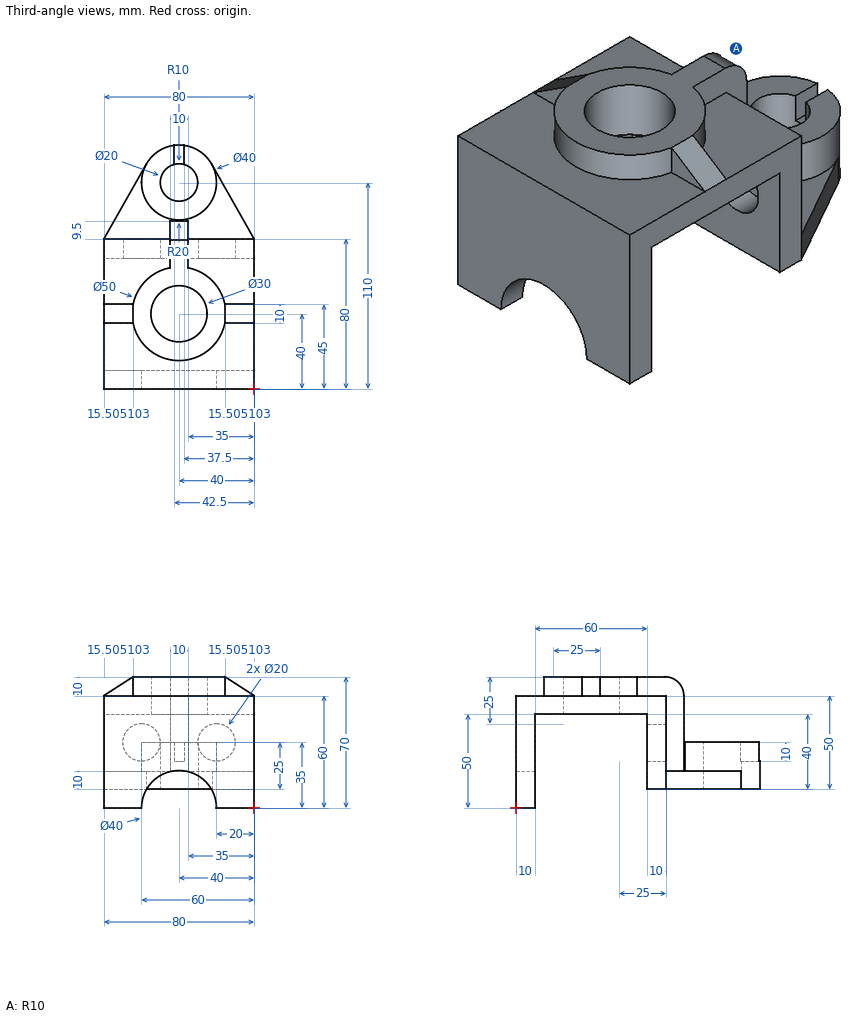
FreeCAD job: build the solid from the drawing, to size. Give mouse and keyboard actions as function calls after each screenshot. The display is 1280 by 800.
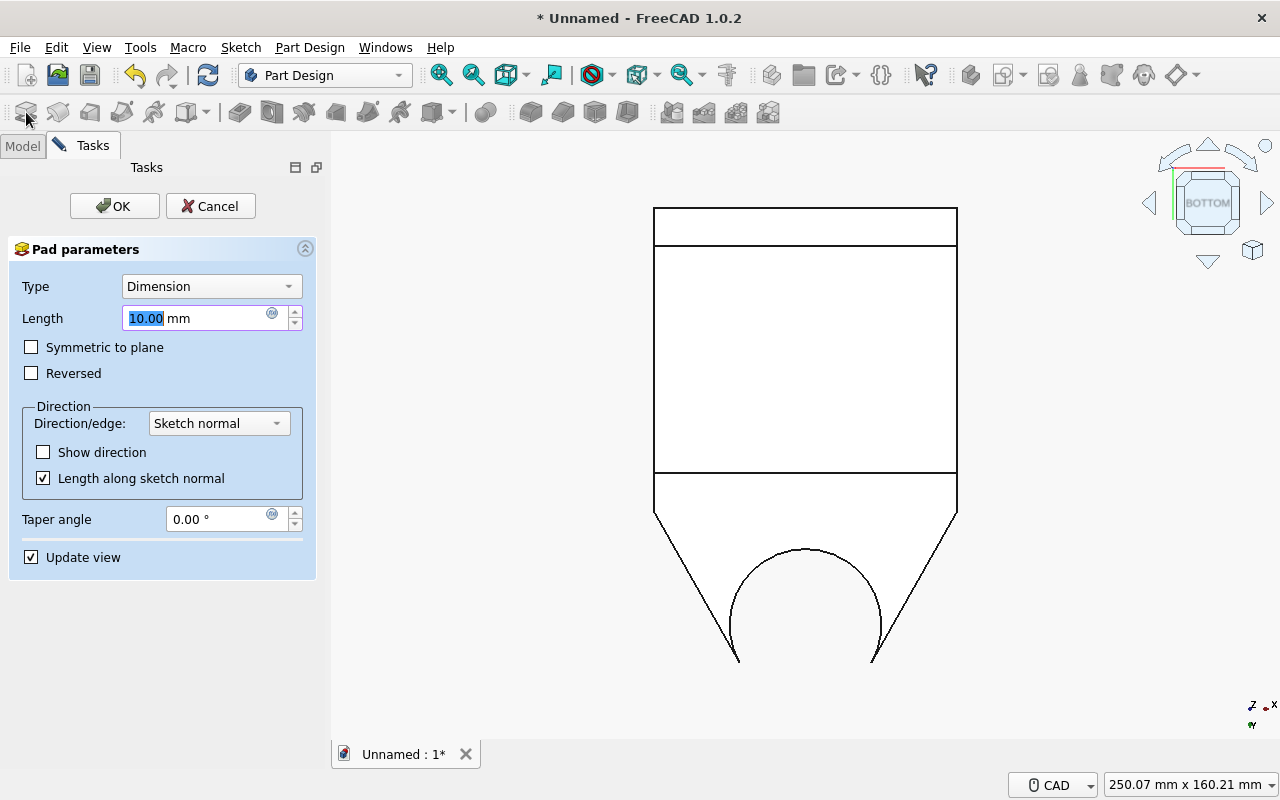
text(25)
key(Tab)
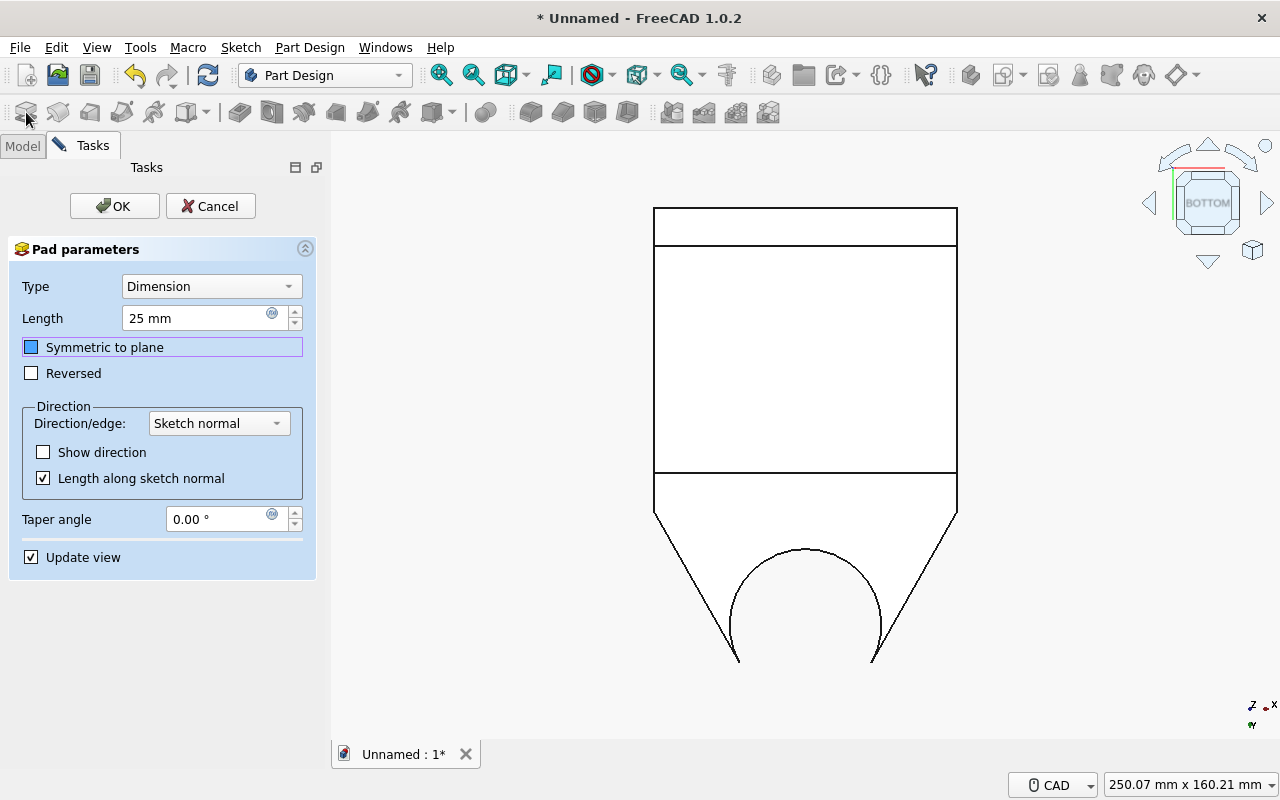
click(30, 373)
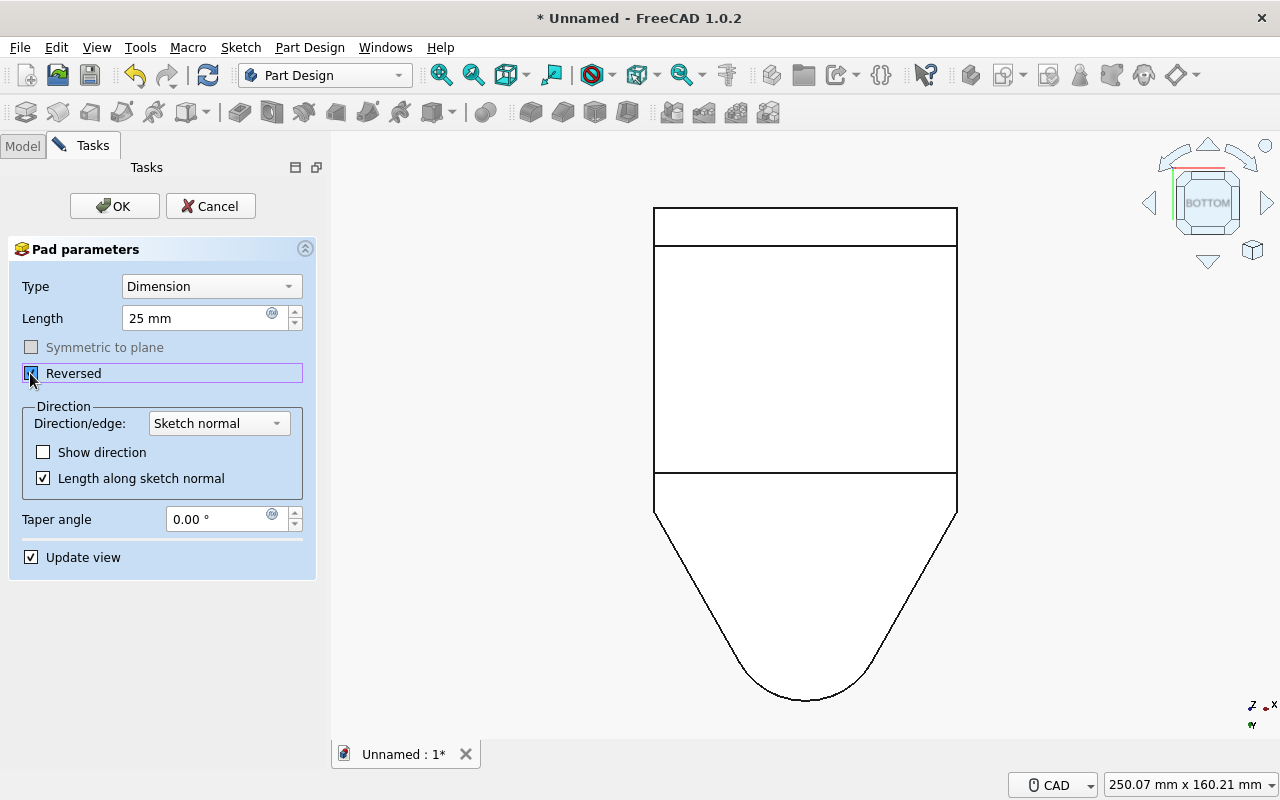
click(115, 206)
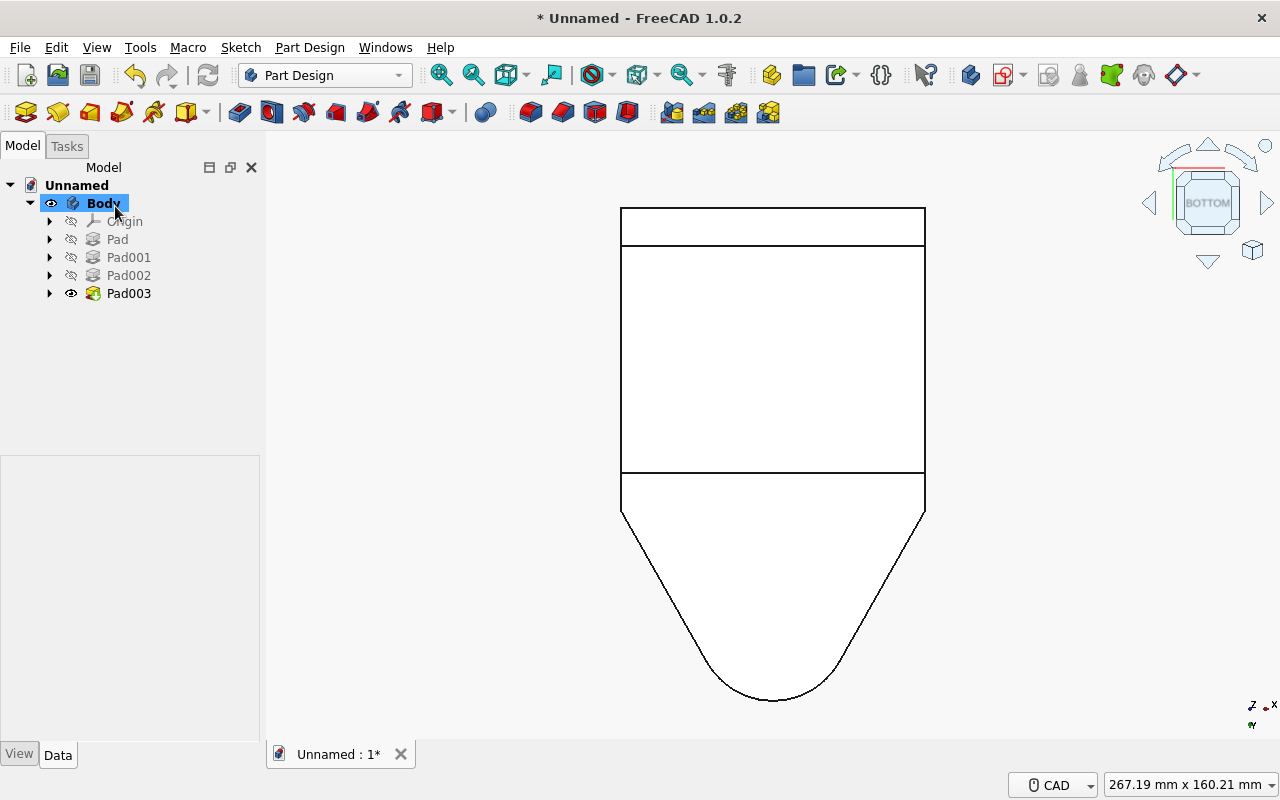
key(0)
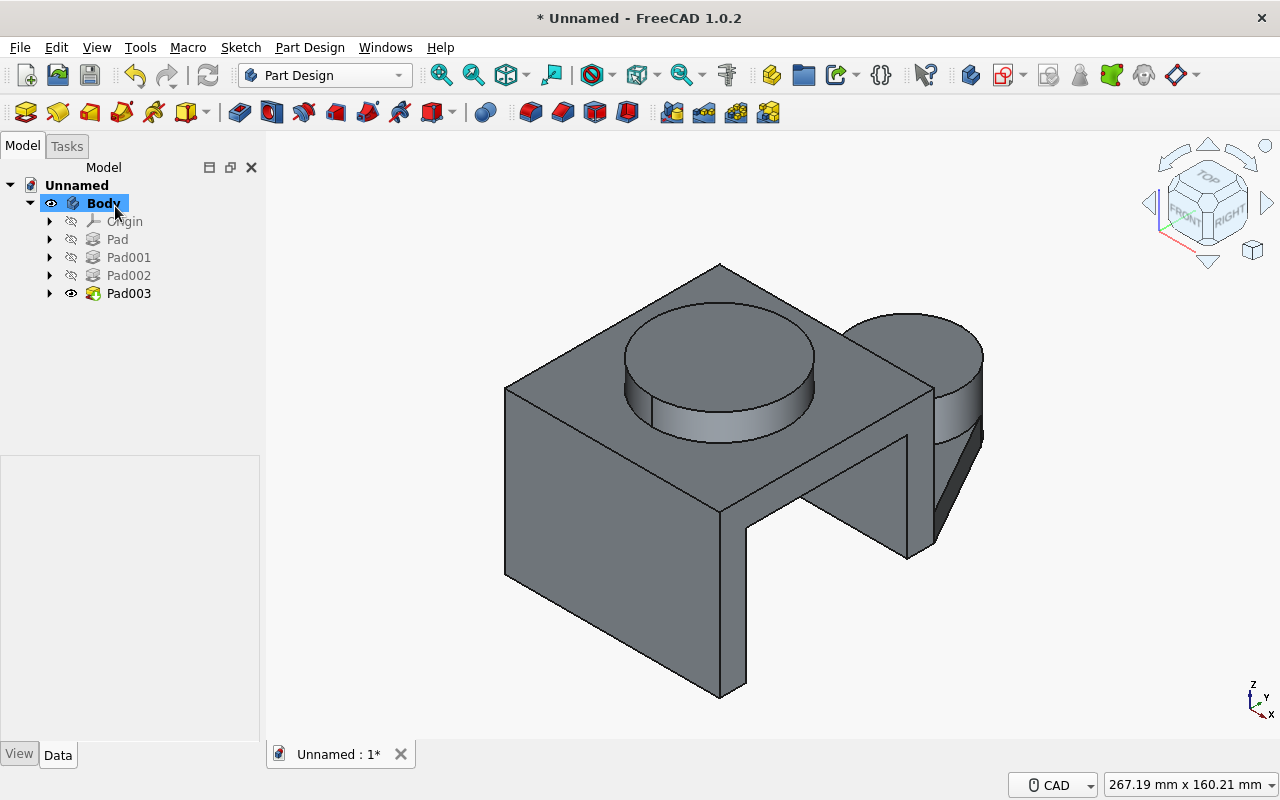
click(720, 356)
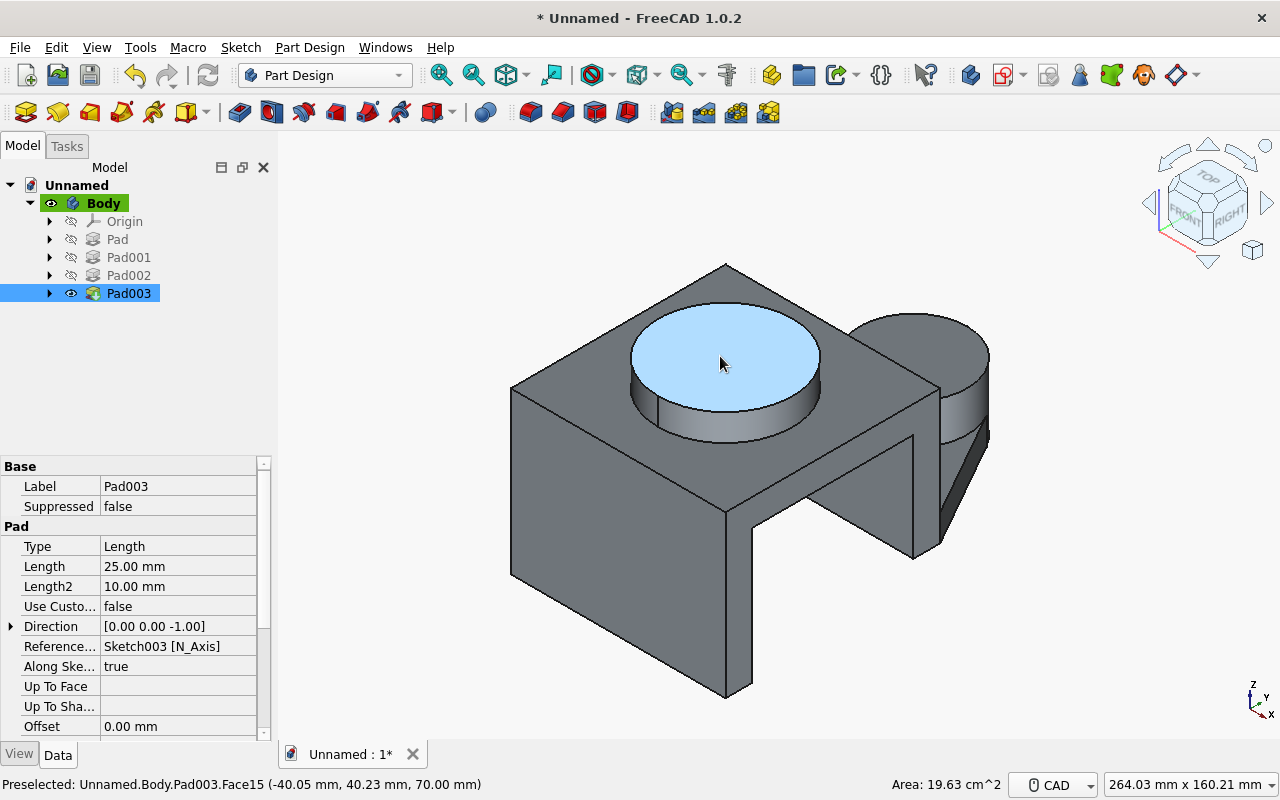
click(1004, 76)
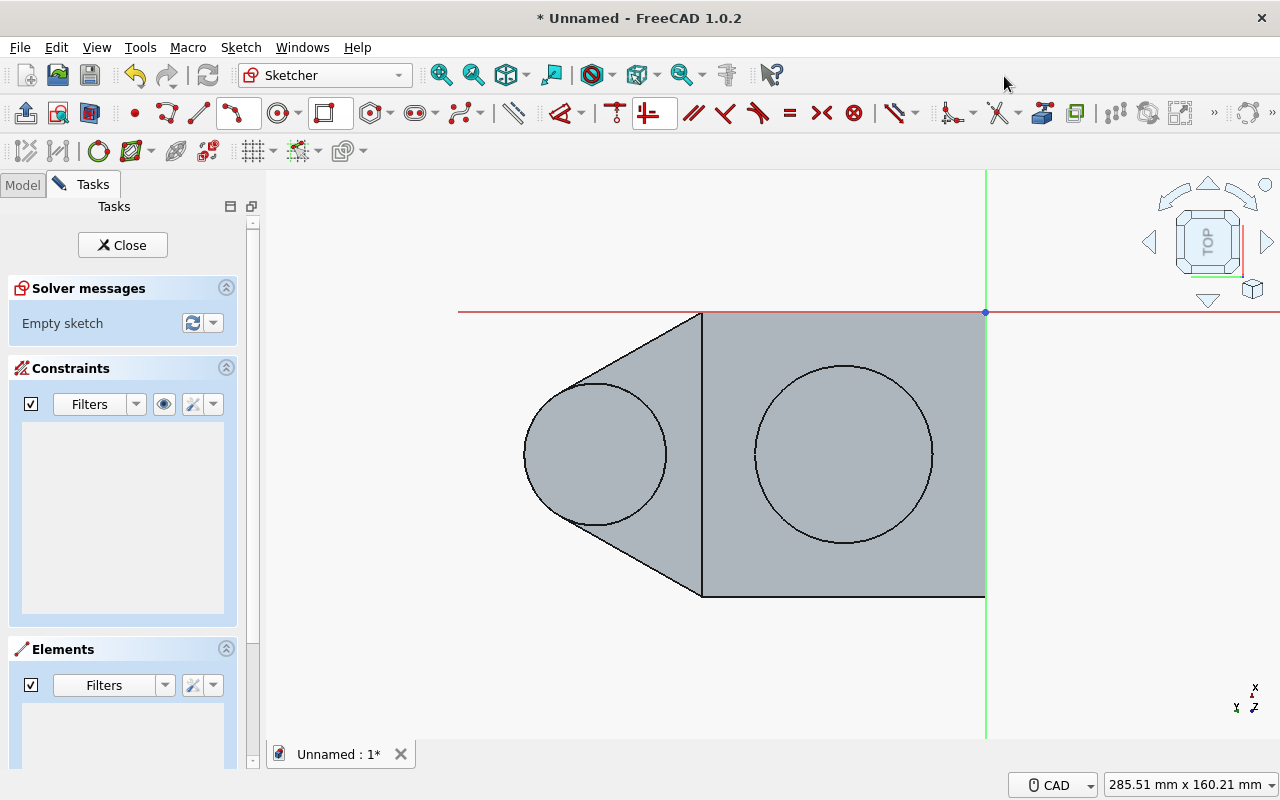
scroll(683, 455, up, 12)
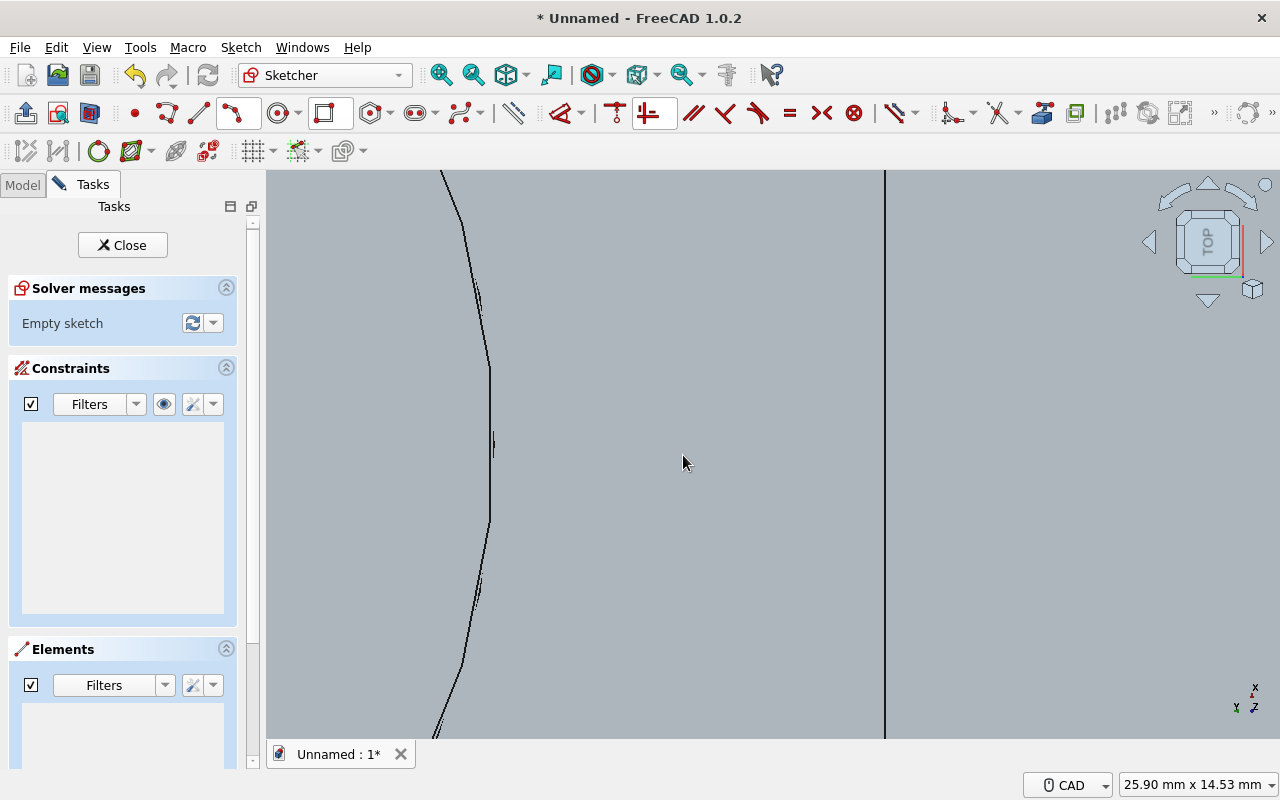
click(324, 114)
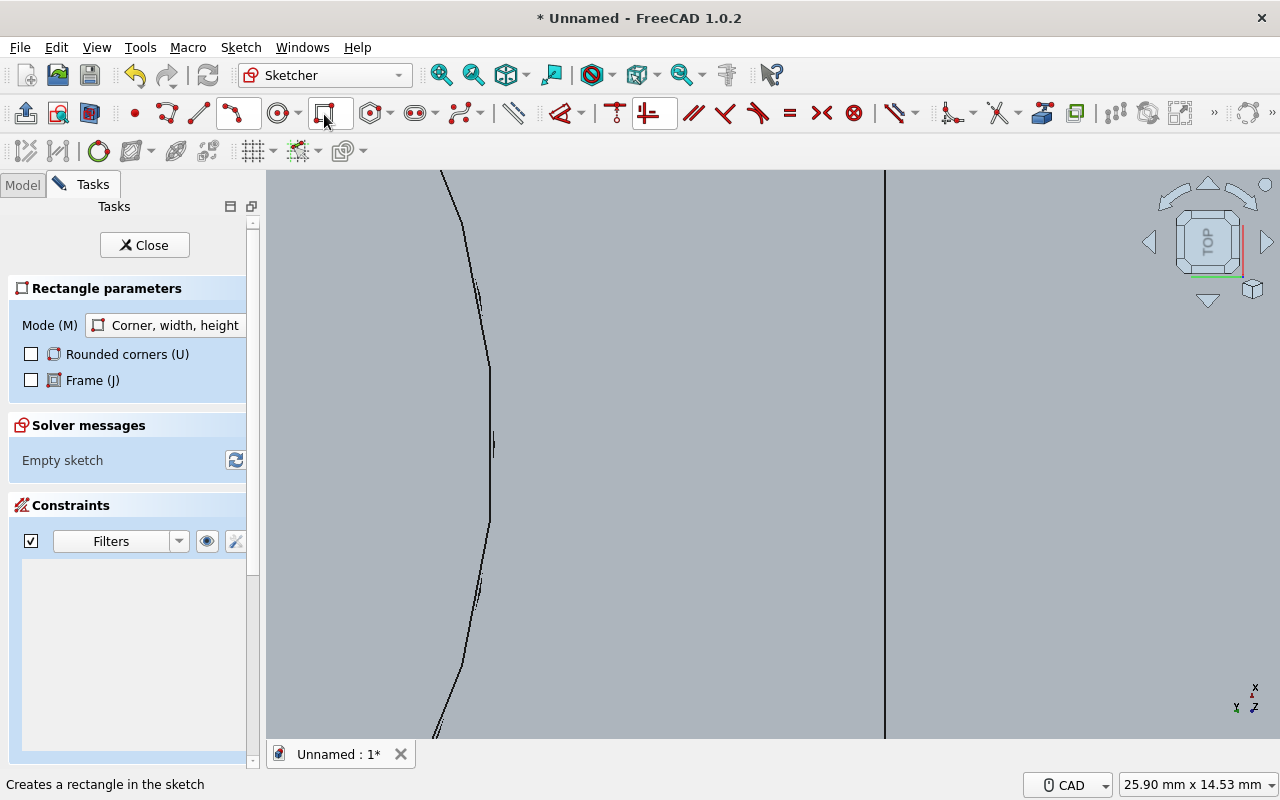
click(513, 249)
move(885, 640)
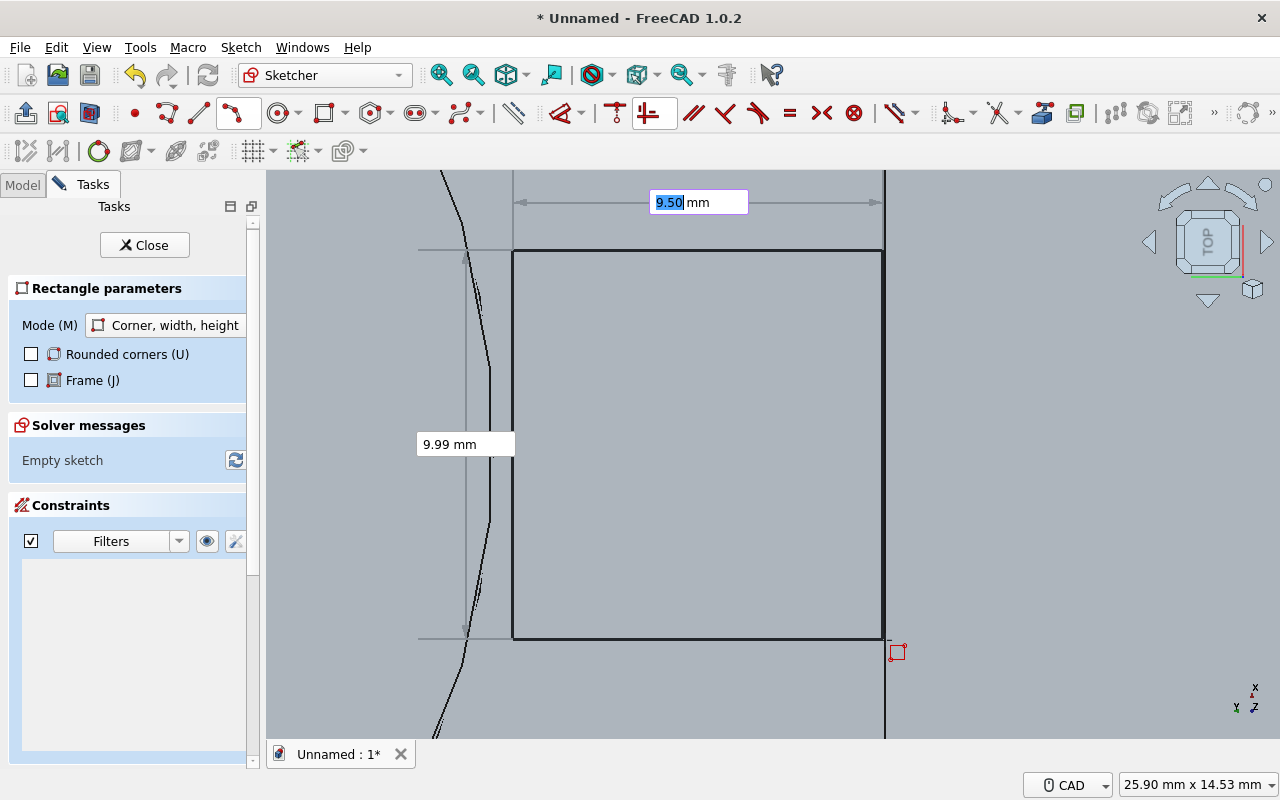
text(9.5)
key(Tab)
text(10)
key(Return)
key(Escape)